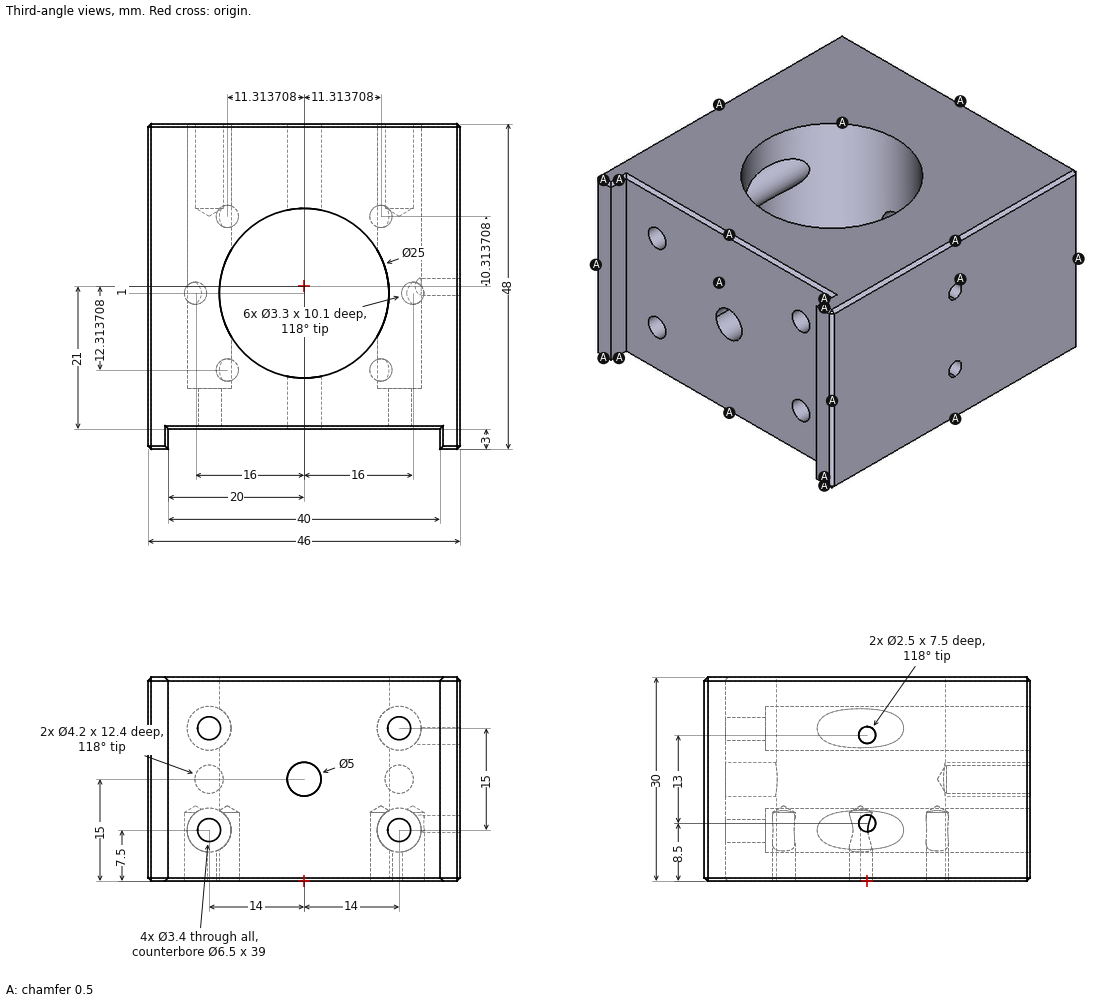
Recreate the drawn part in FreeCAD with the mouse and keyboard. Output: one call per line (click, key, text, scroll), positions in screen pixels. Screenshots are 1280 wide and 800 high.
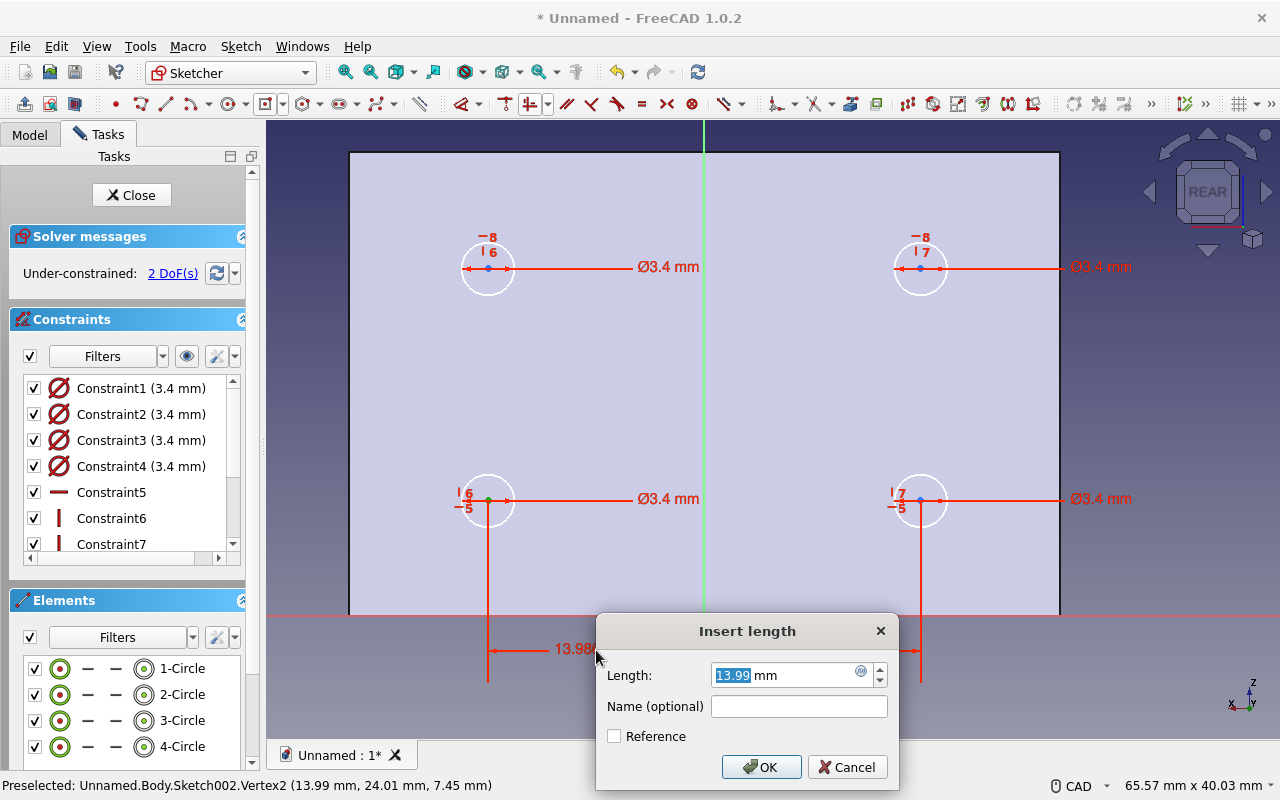
text(14)
key(Return)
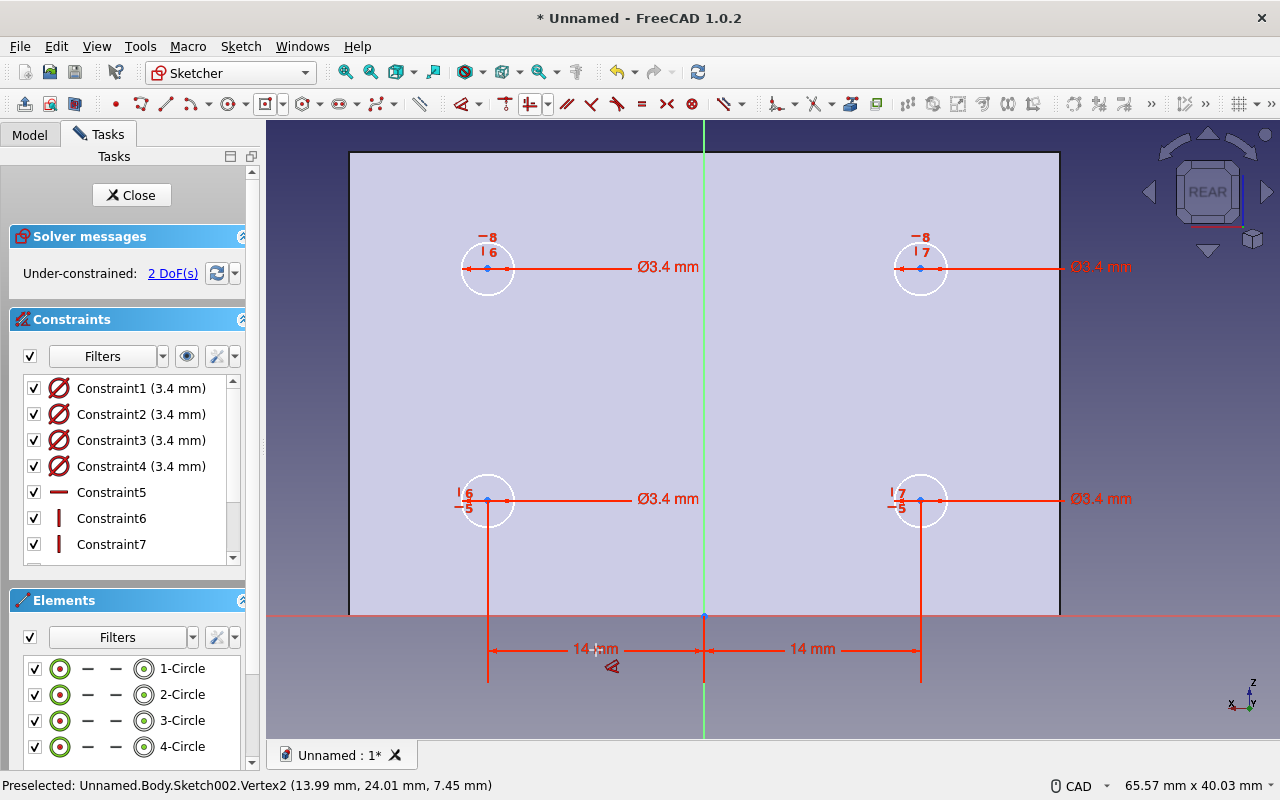
click(921, 501)
click(955, 559)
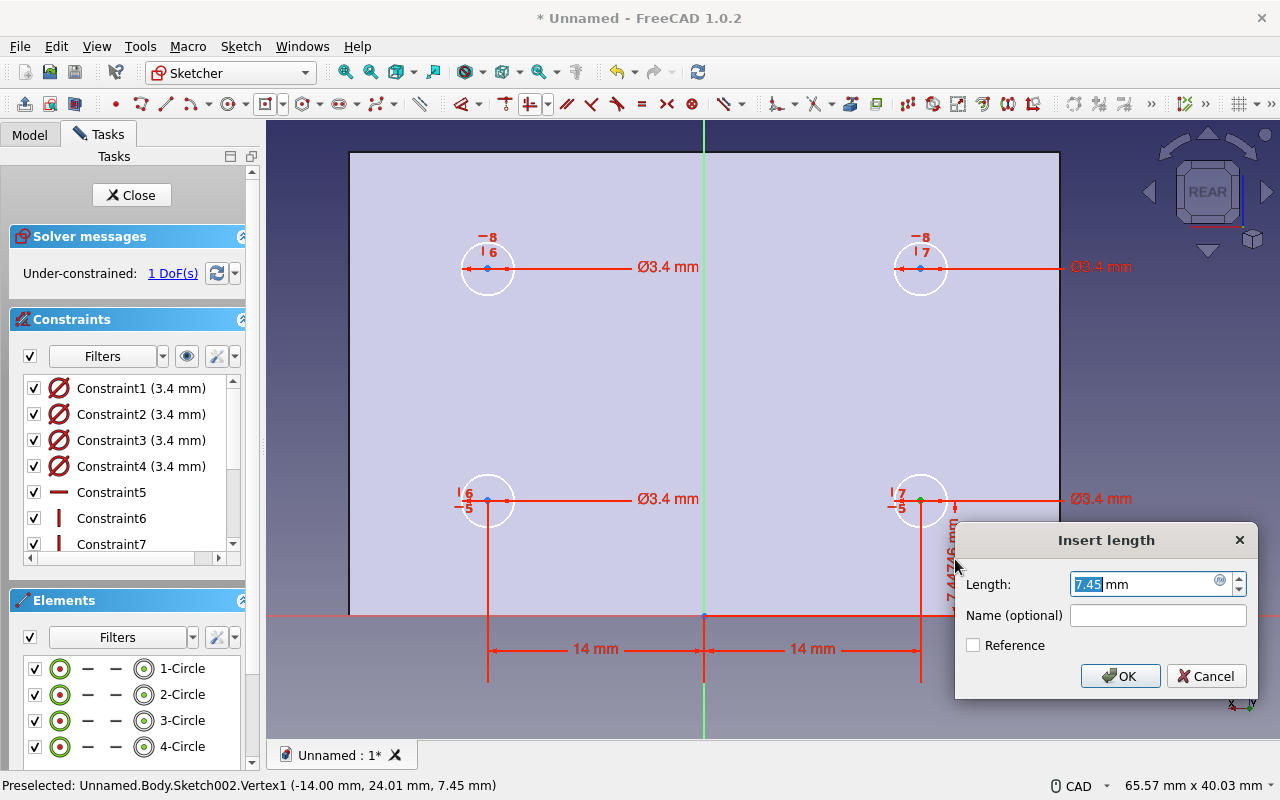
text(7.5)
key(Return)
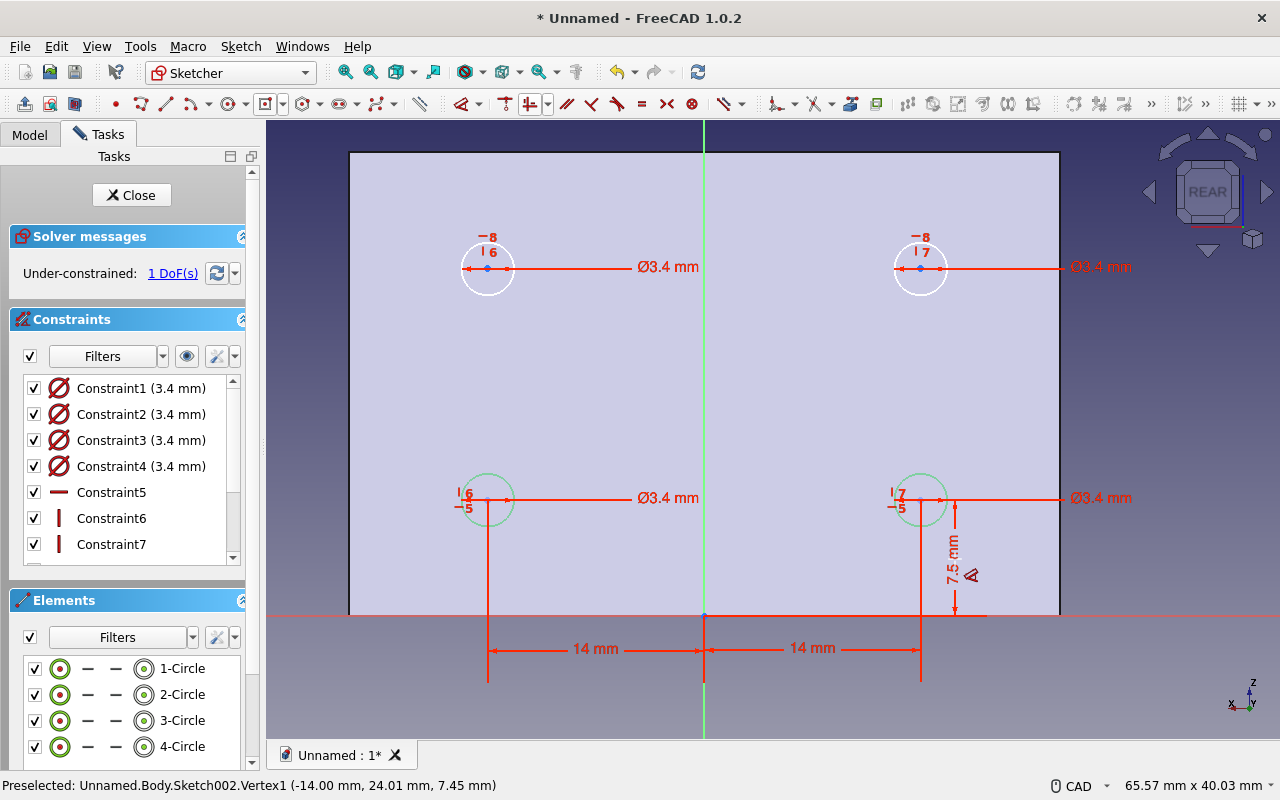
click(488, 500)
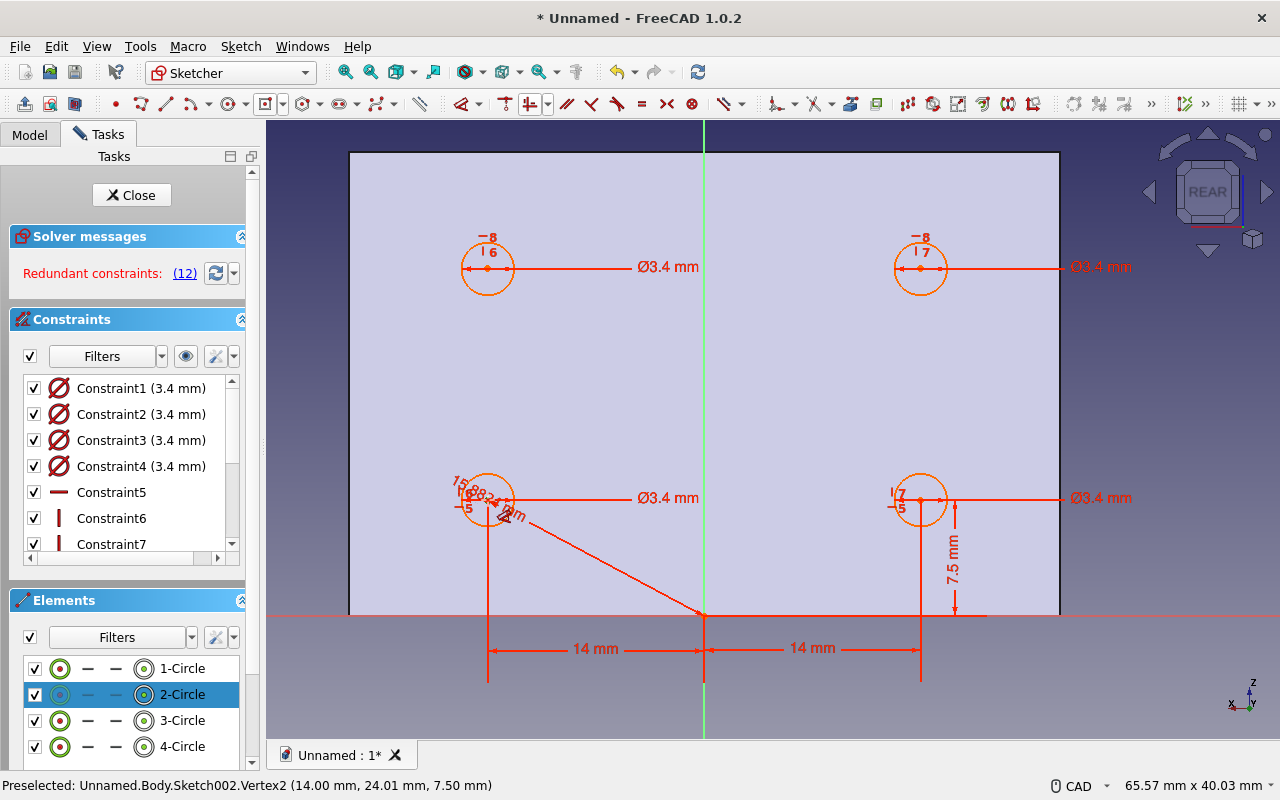
click(488, 269)
click(454, 385)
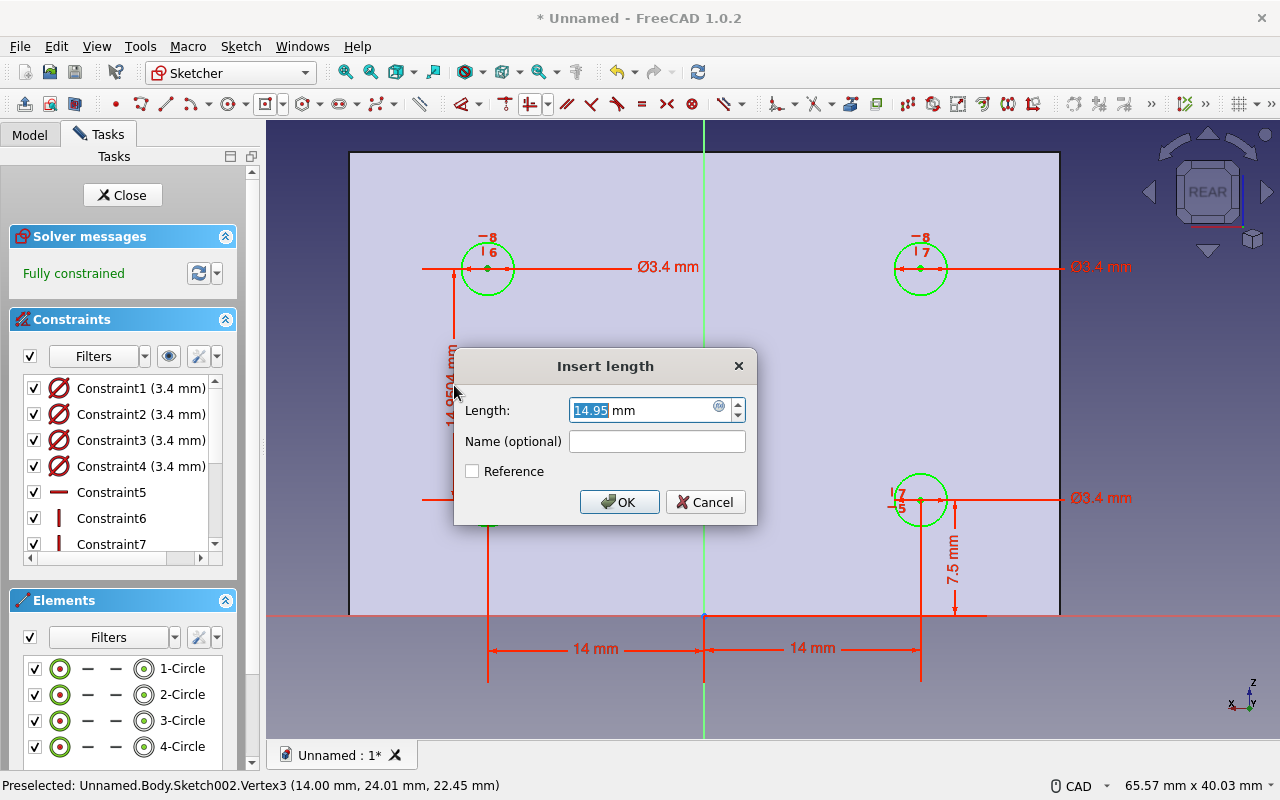
text(15)
key(Return)
key(Escape)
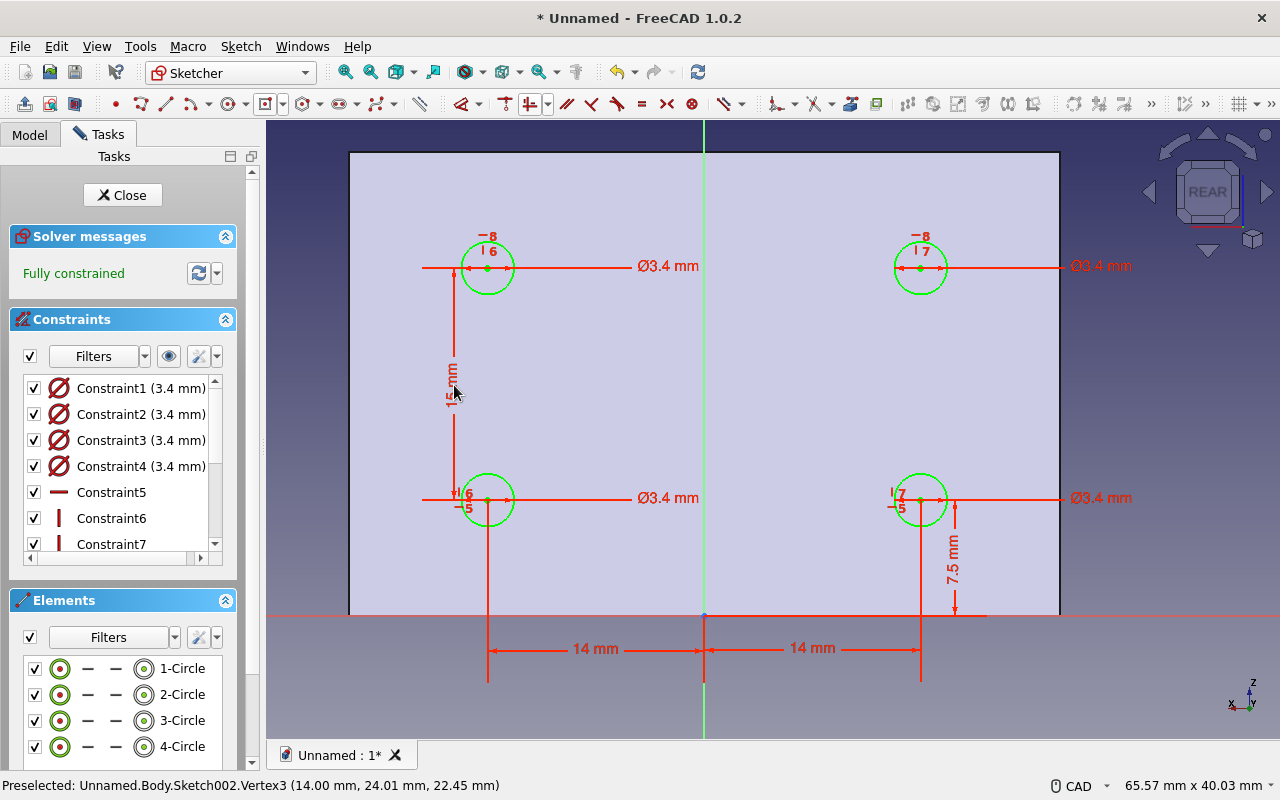
click(123, 195)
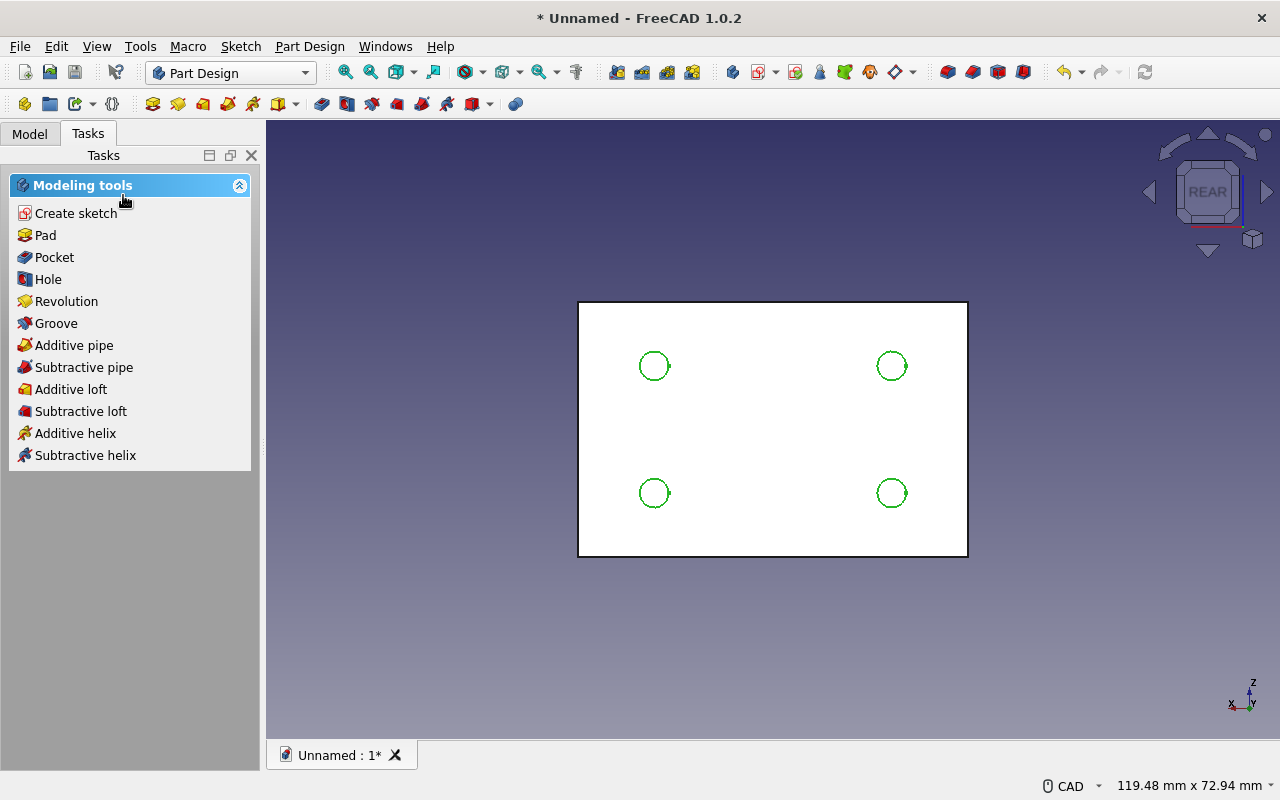
click(347, 104)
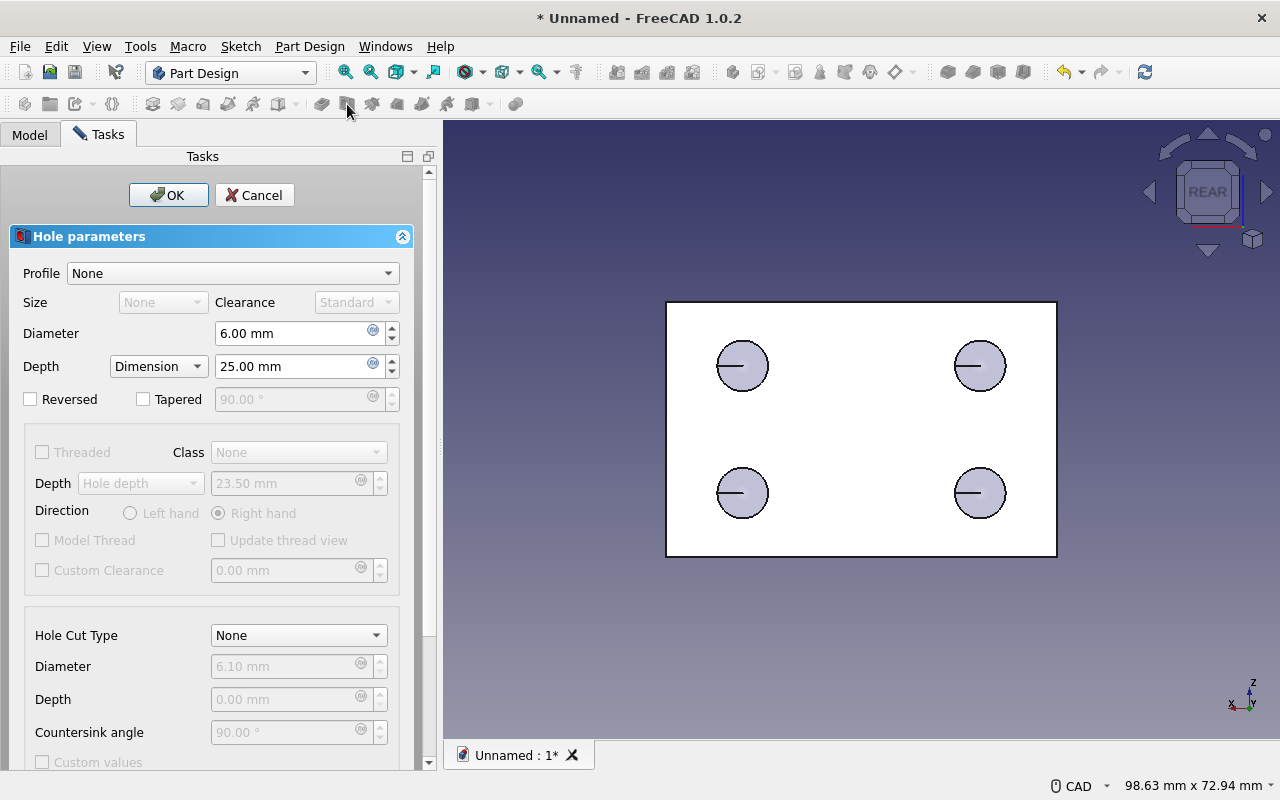
triple_click(300, 334)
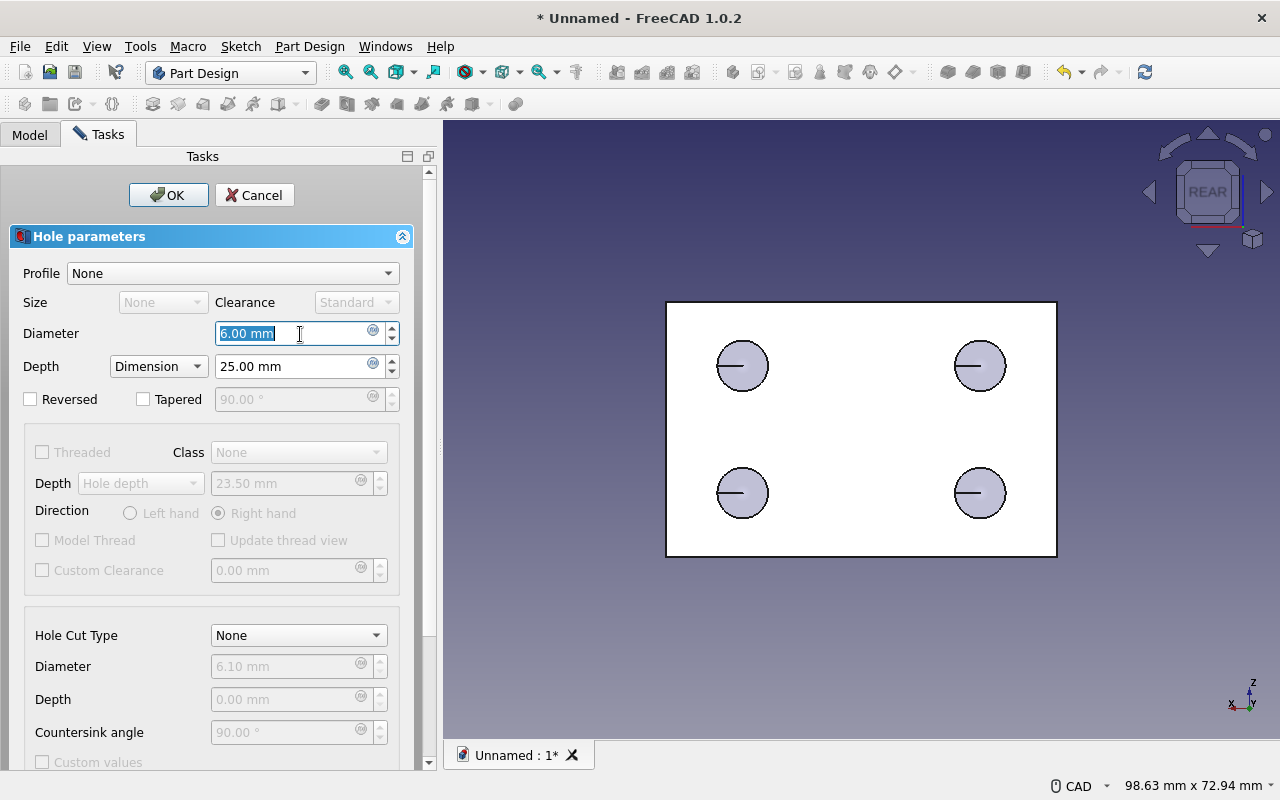
text(3.4)
key(Tab)